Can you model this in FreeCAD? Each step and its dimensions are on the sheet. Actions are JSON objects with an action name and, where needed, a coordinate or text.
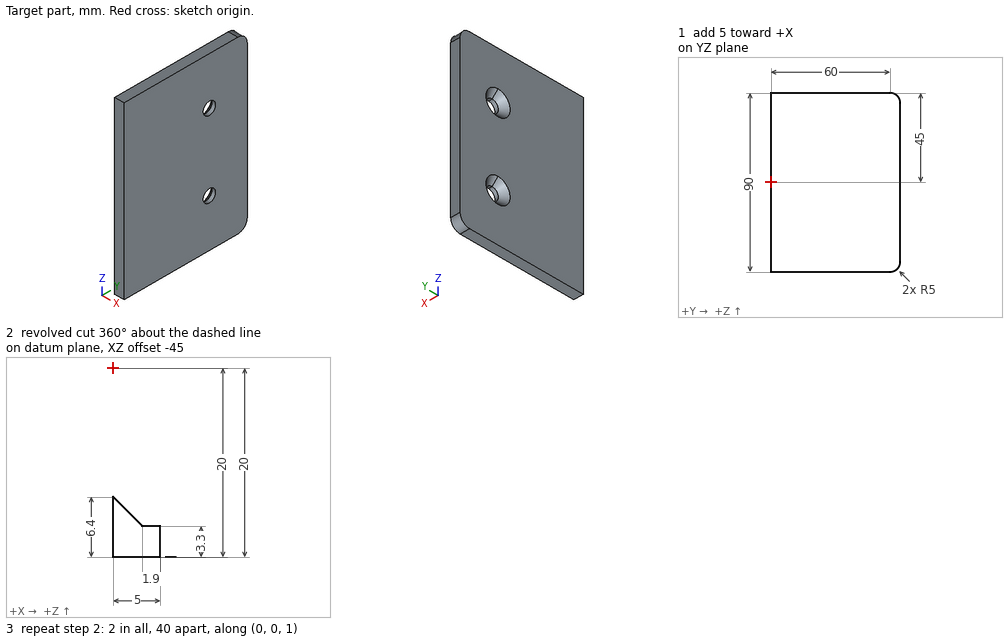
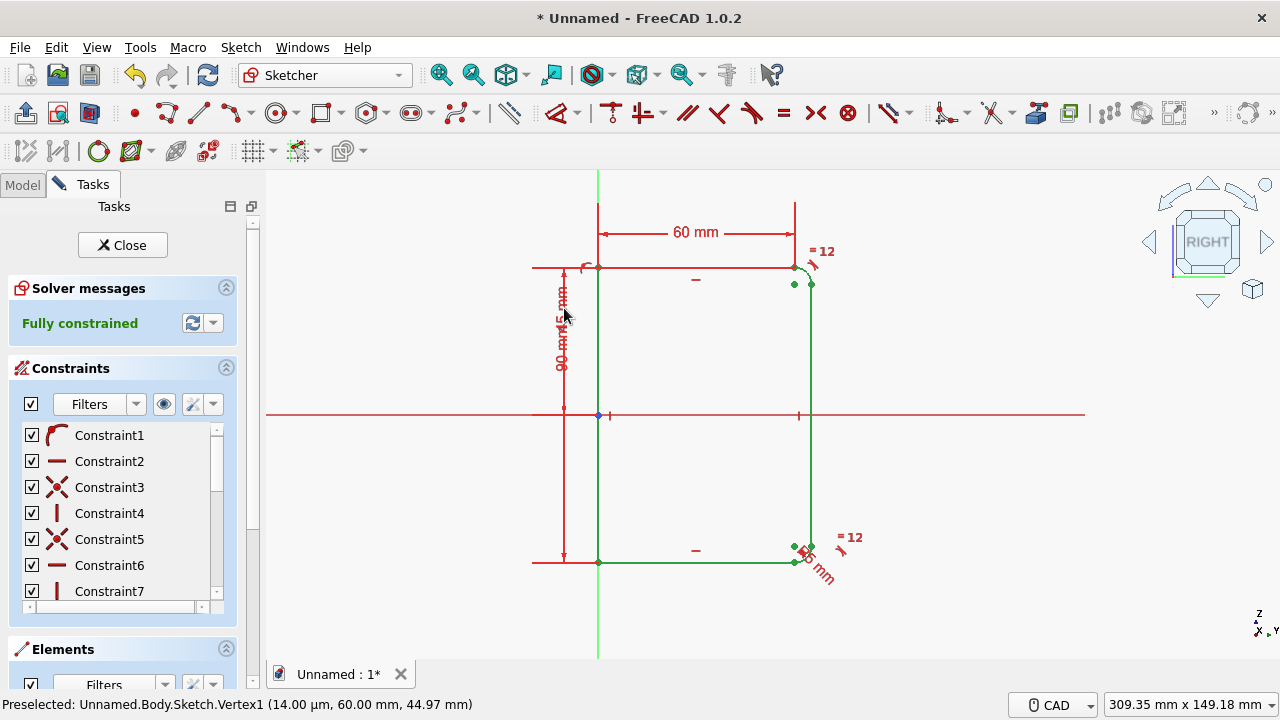
{"action": "left_click", "coordinate": [123, 245]}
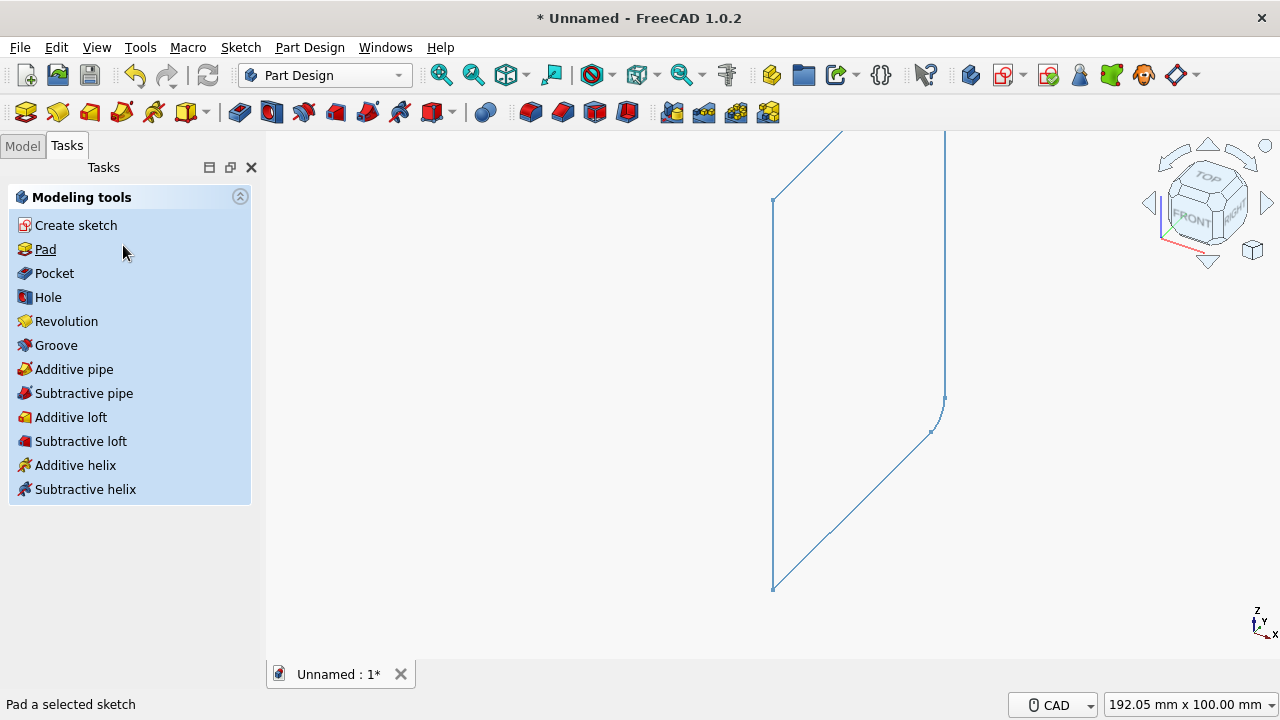
{"action": "left_click", "coordinate": [26, 112]}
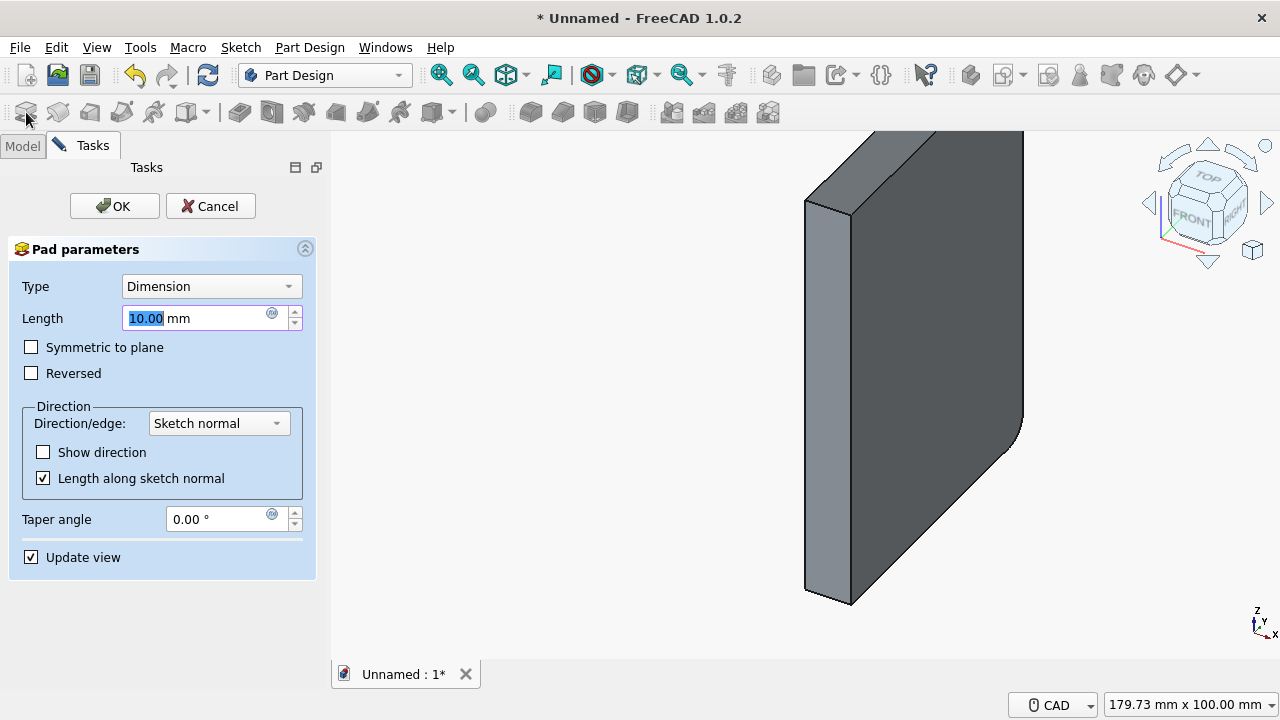
{"action": "type", "text": "5"}
{"action": "key", "text": "Tab"}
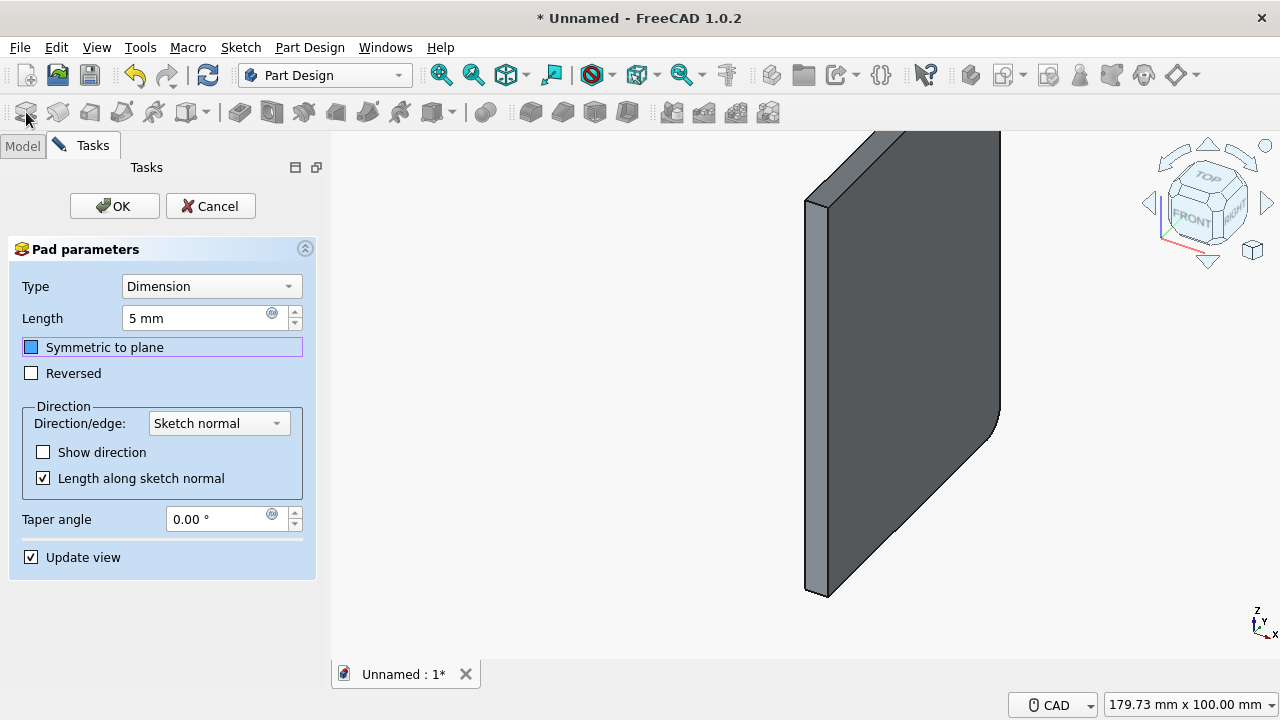
{"action": "left_click", "coordinate": [115, 206]}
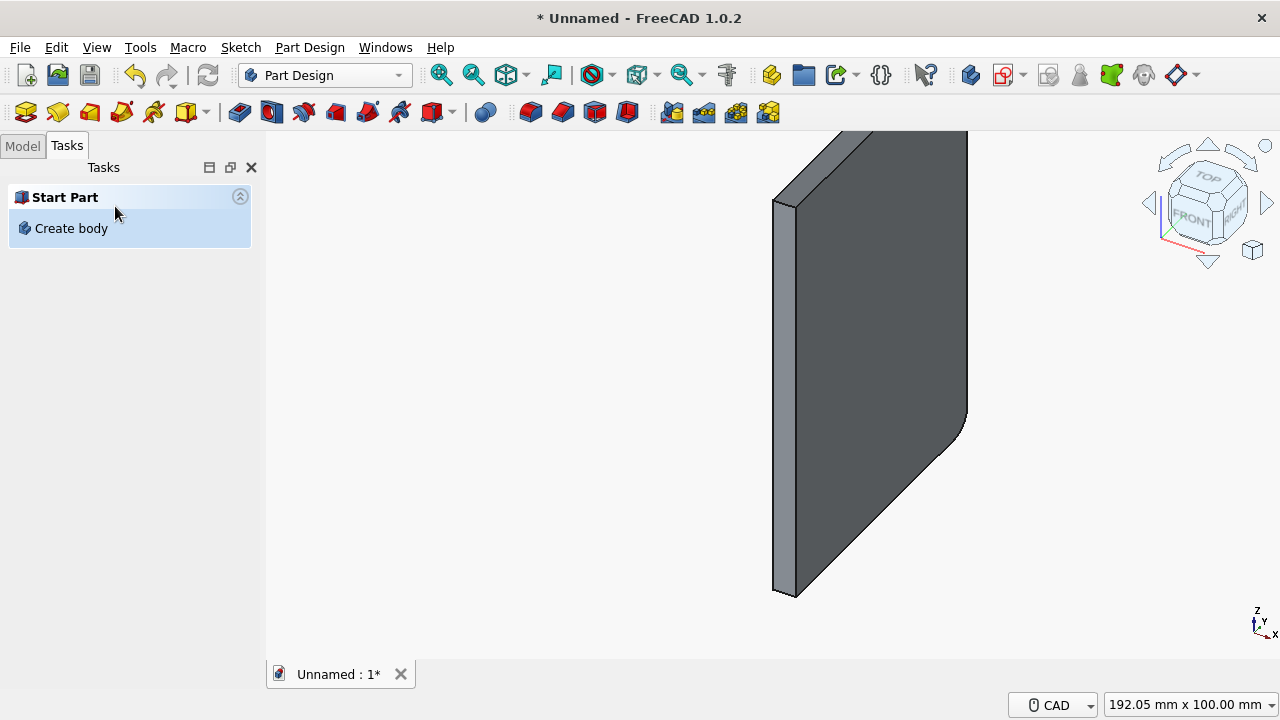
{"action": "left_click", "coordinate": [442, 76]}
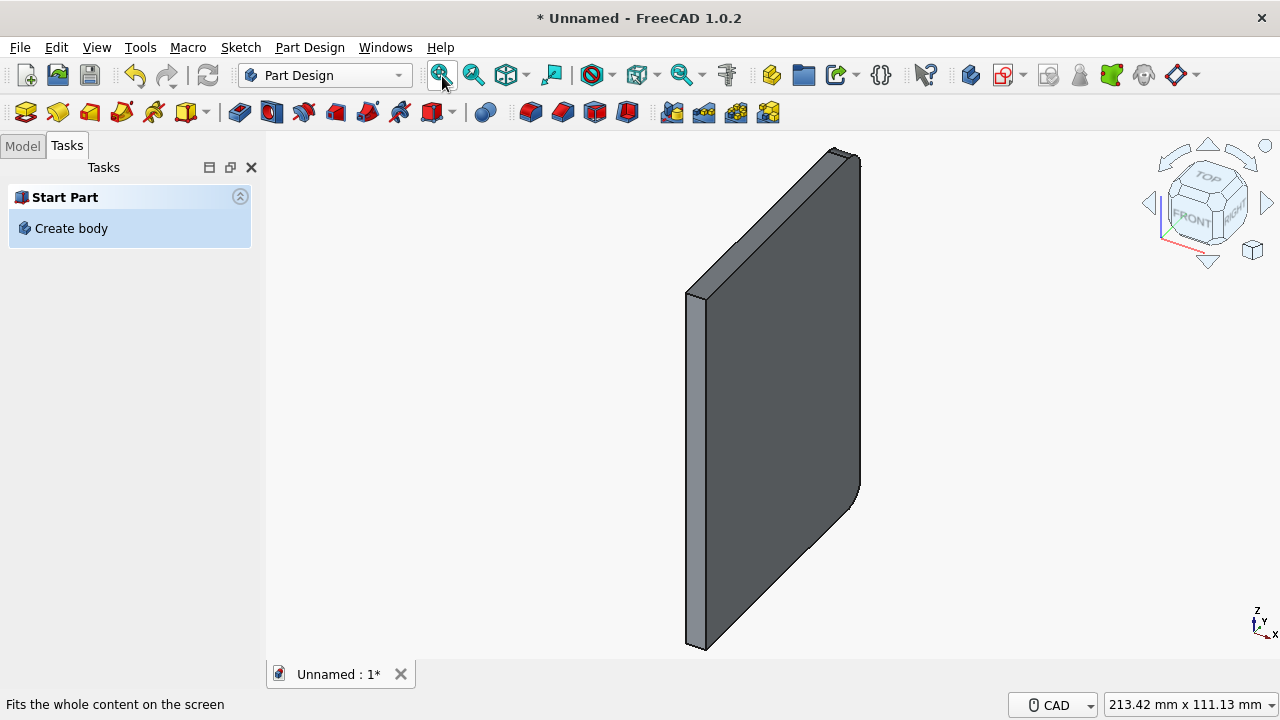
{"action": "left_click", "coordinate": [23, 145]}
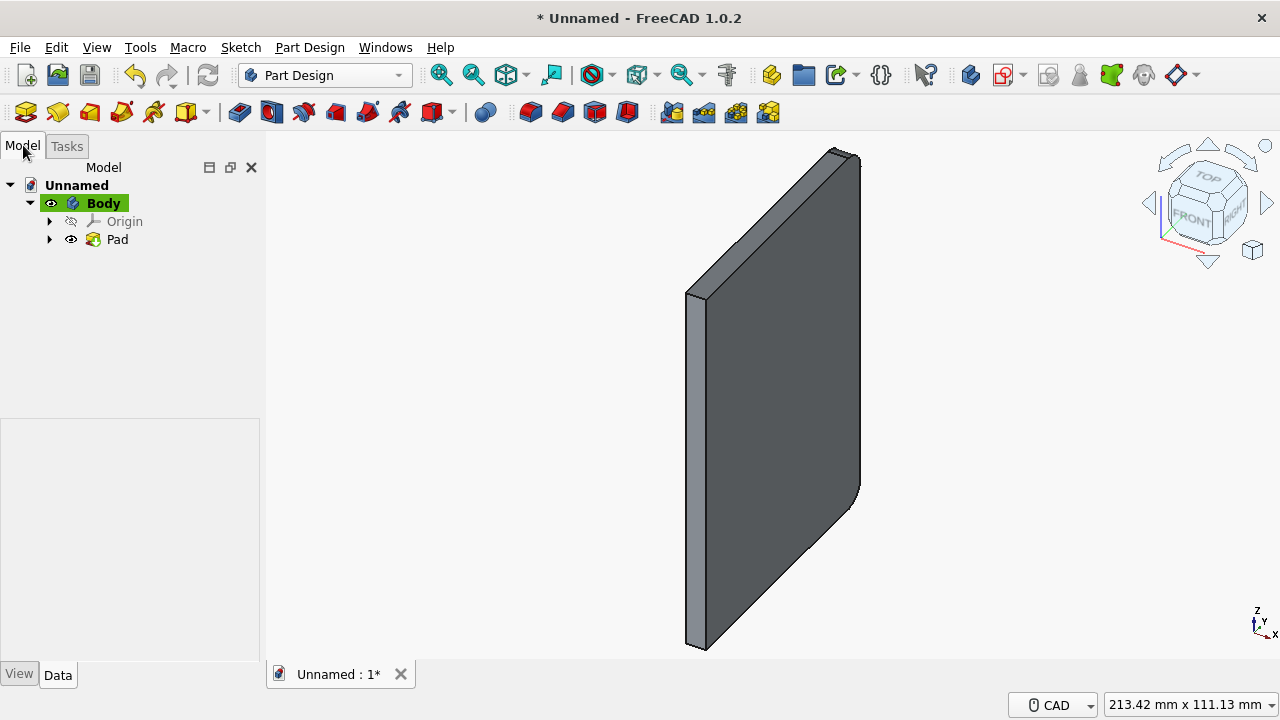
{"action": "left_click", "coordinate": [50, 221]}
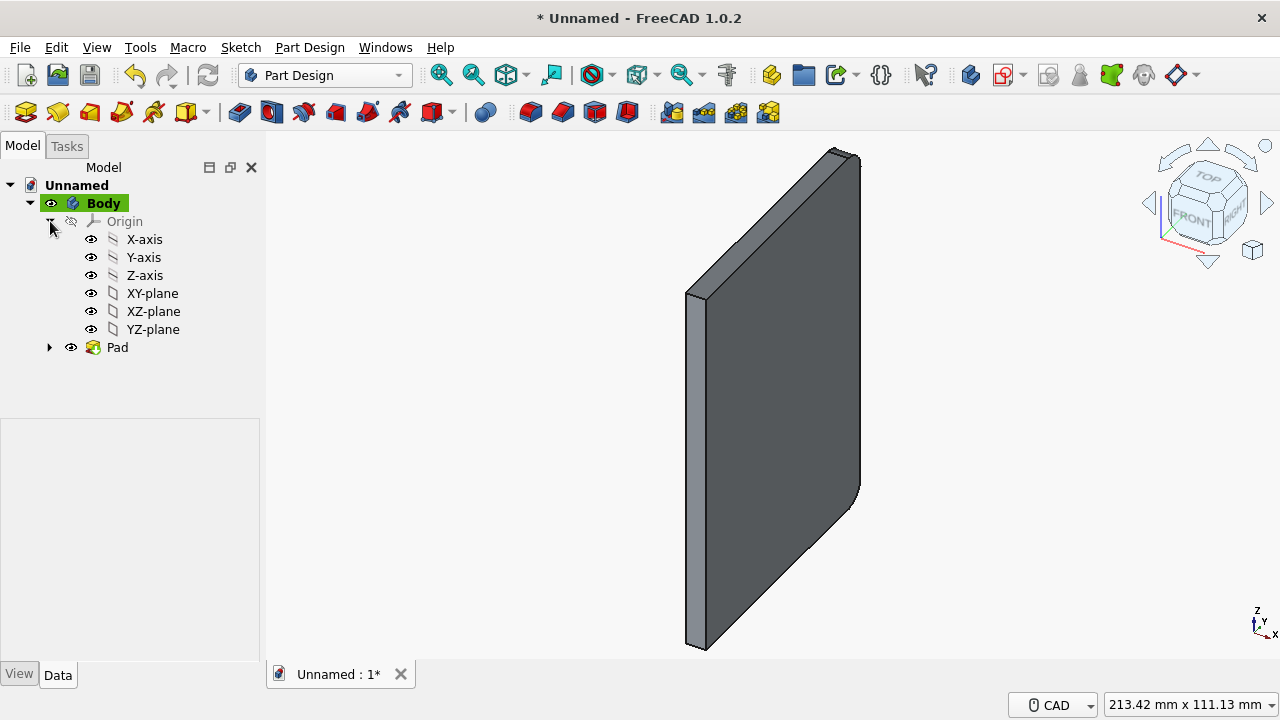
{"action": "left_click", "coordinate": [136, 311]}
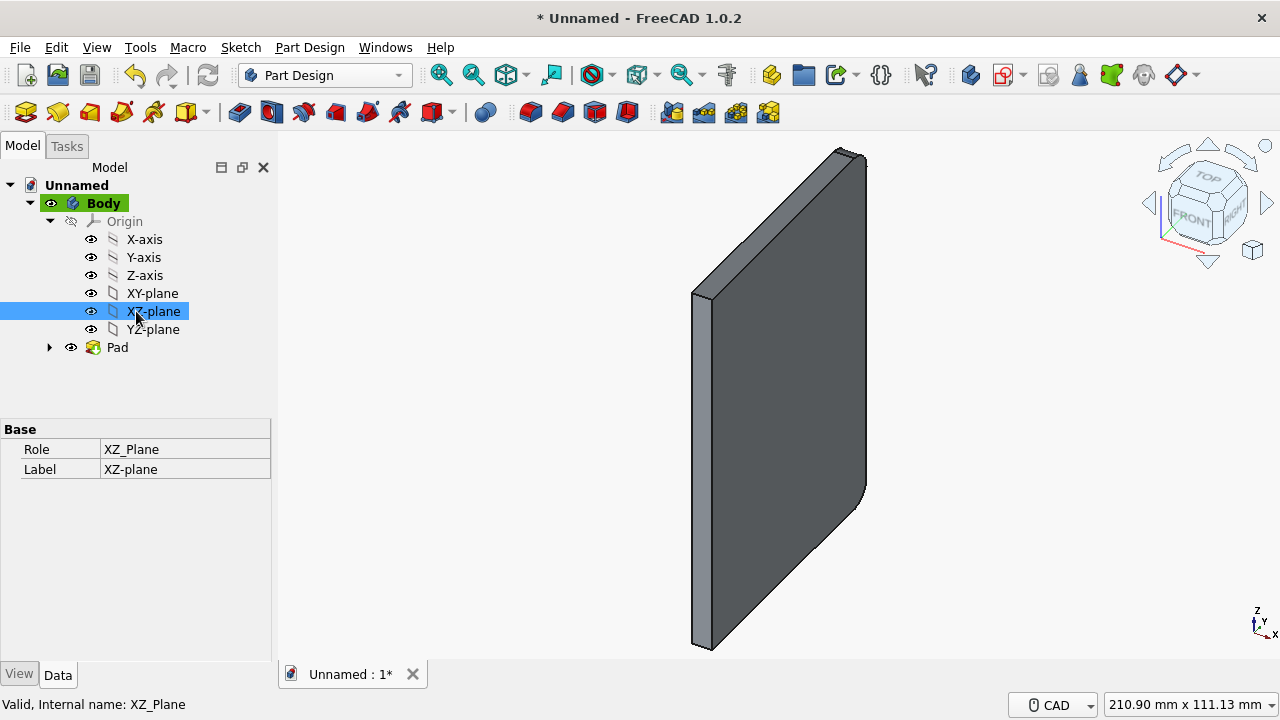
{"action": "left_click", "coordinate": [1176, 76]}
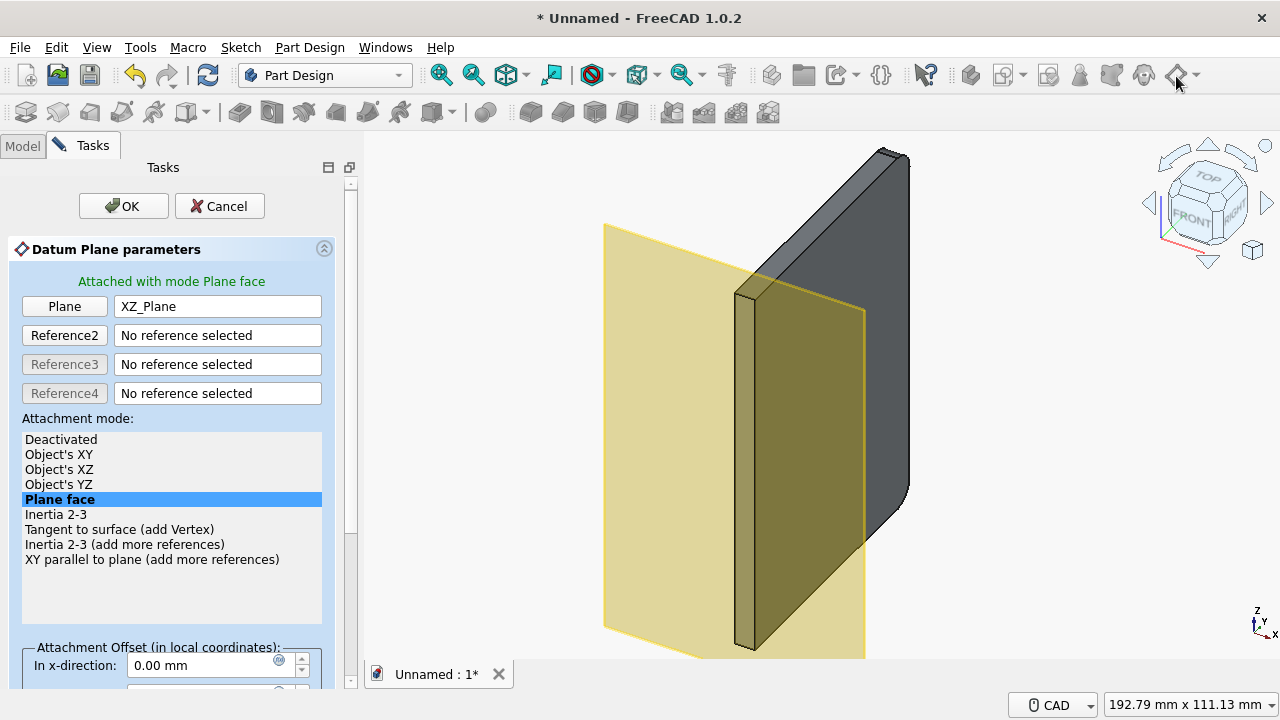
{"action": "scroll", "coordinate": [351, 432], "scroll_direction": "down", "scroll_amount": 2}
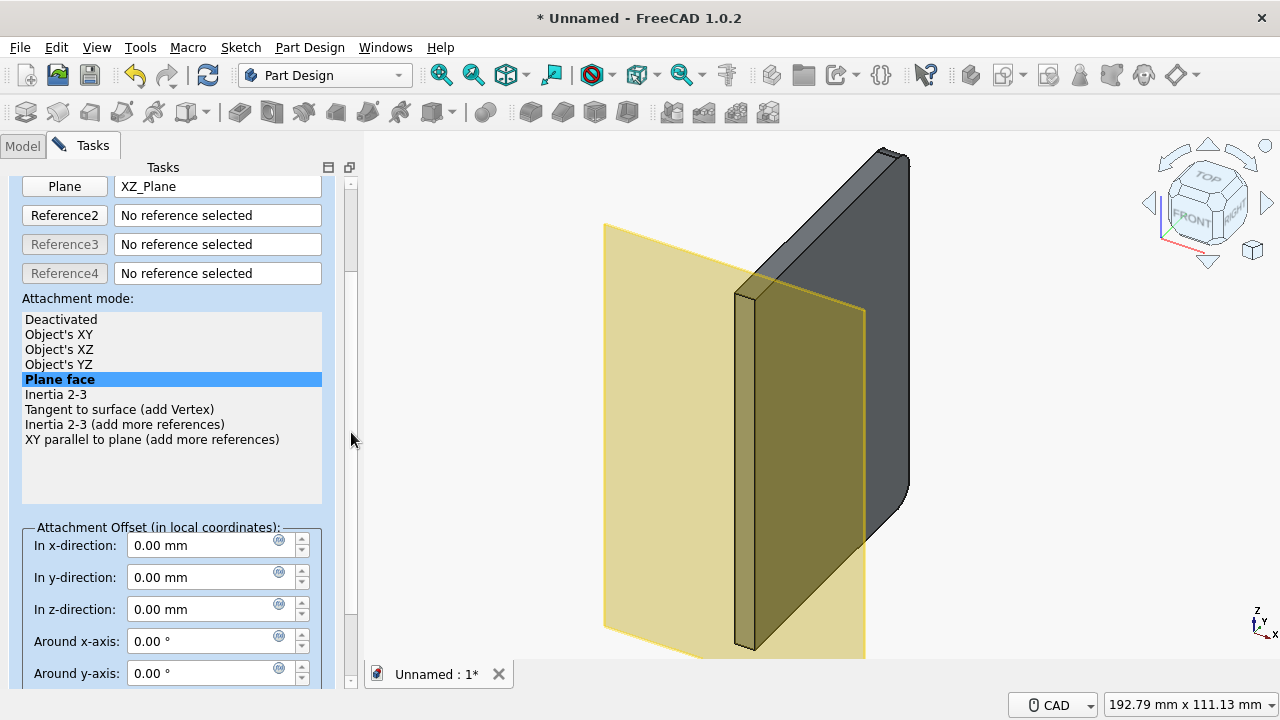
{"action": "triple_click", "coordinate": [210, 609]}